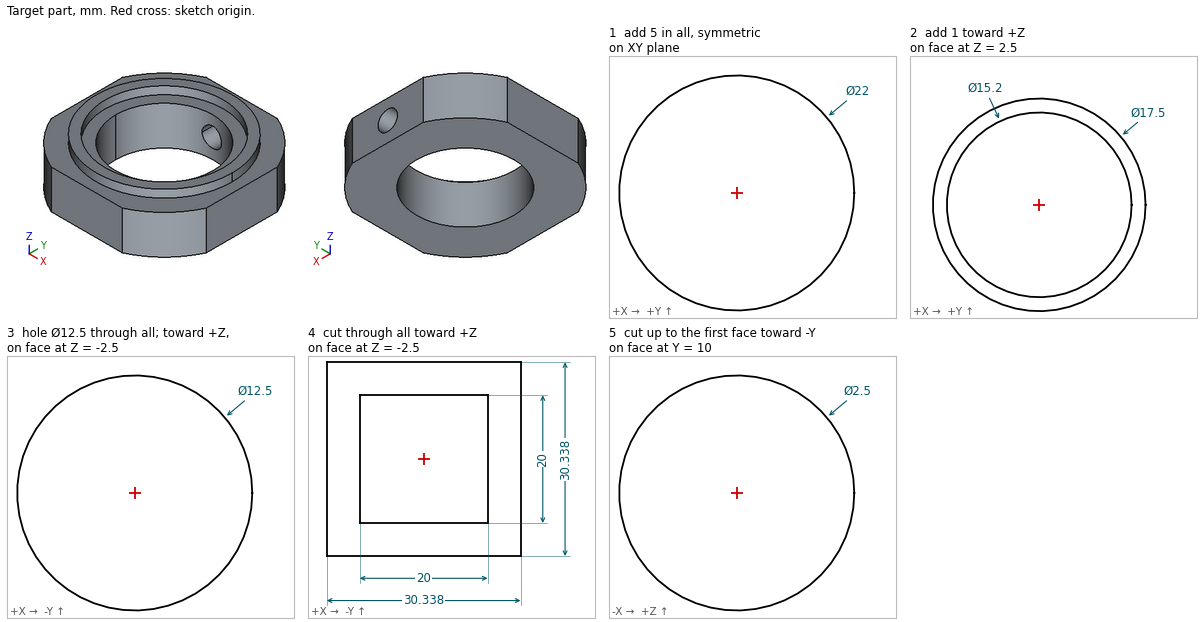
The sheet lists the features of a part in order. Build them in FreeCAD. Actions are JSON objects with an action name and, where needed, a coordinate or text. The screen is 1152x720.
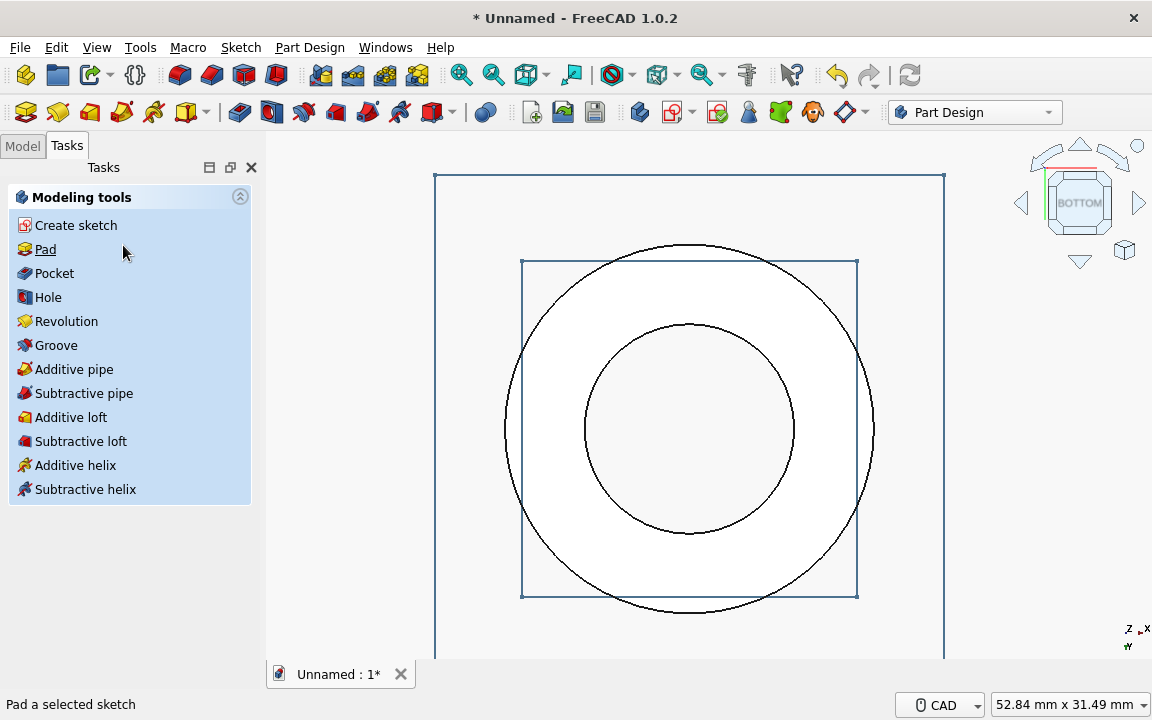
{"action": "left_click", "coordinate": [240, 112]}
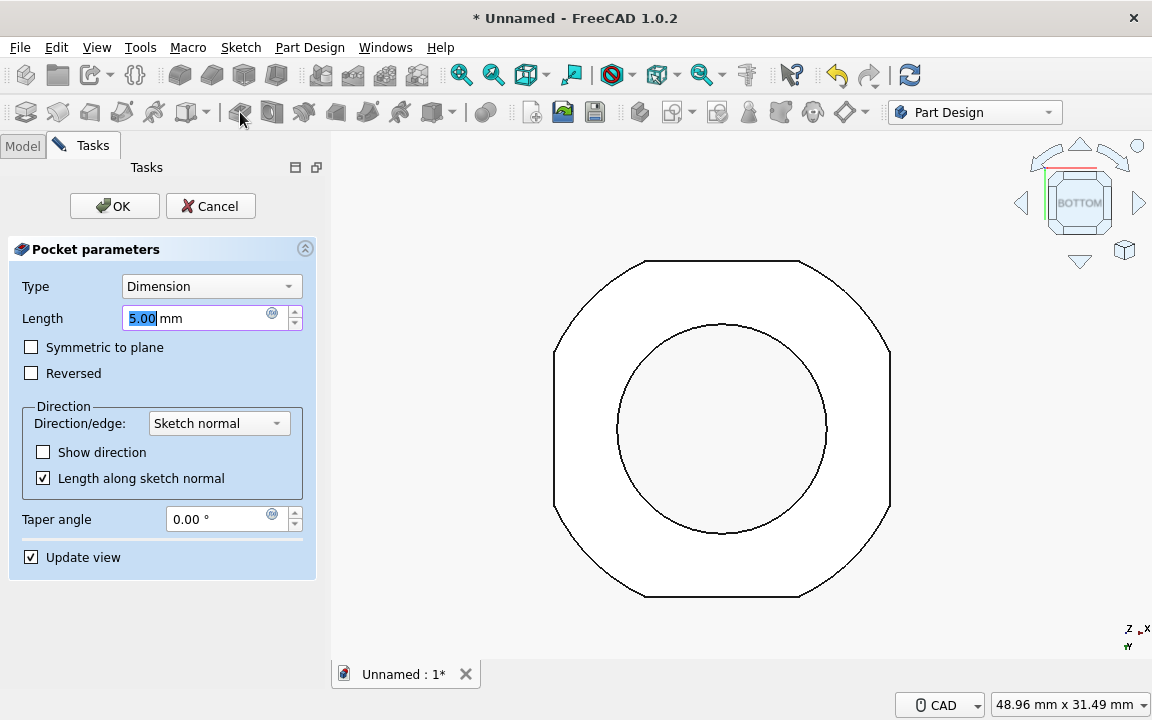
{"action": "left_click", "coordinate": [212, 286]}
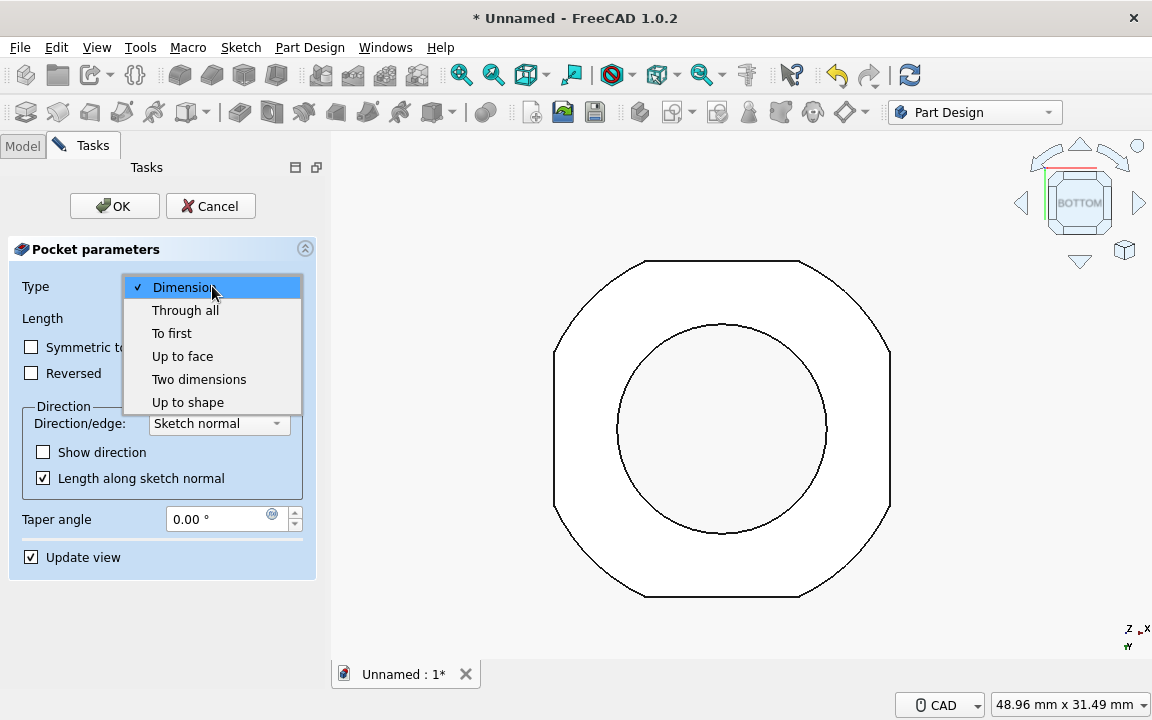
{"action": "left_click", "coordinate": [212, 310]}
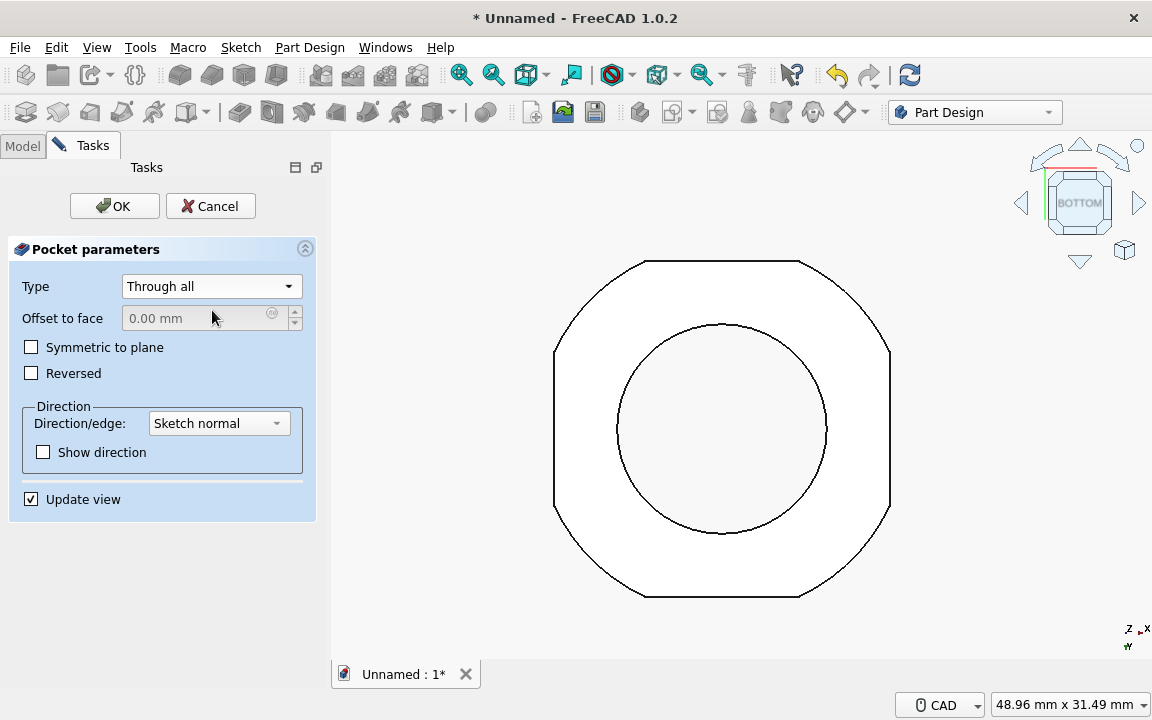
{"action": "left_click", "coordinate": [115, 206]}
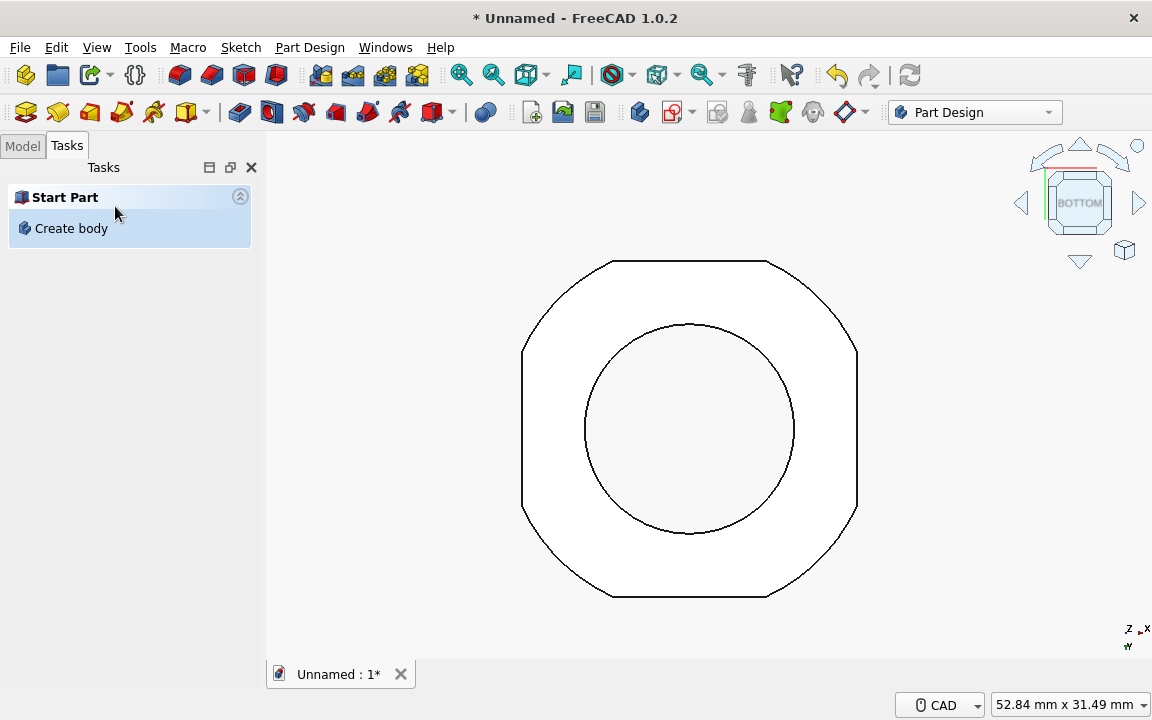
{"action": "key", "text": "4"}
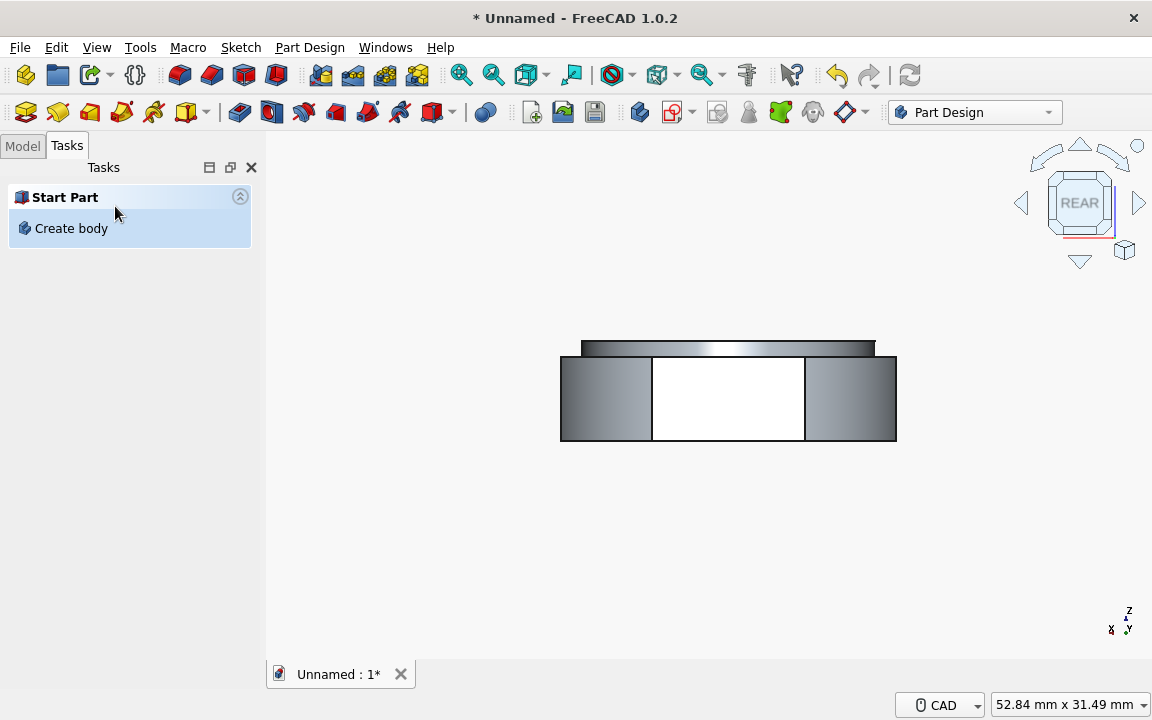
{"action": "key", "text": "v f"}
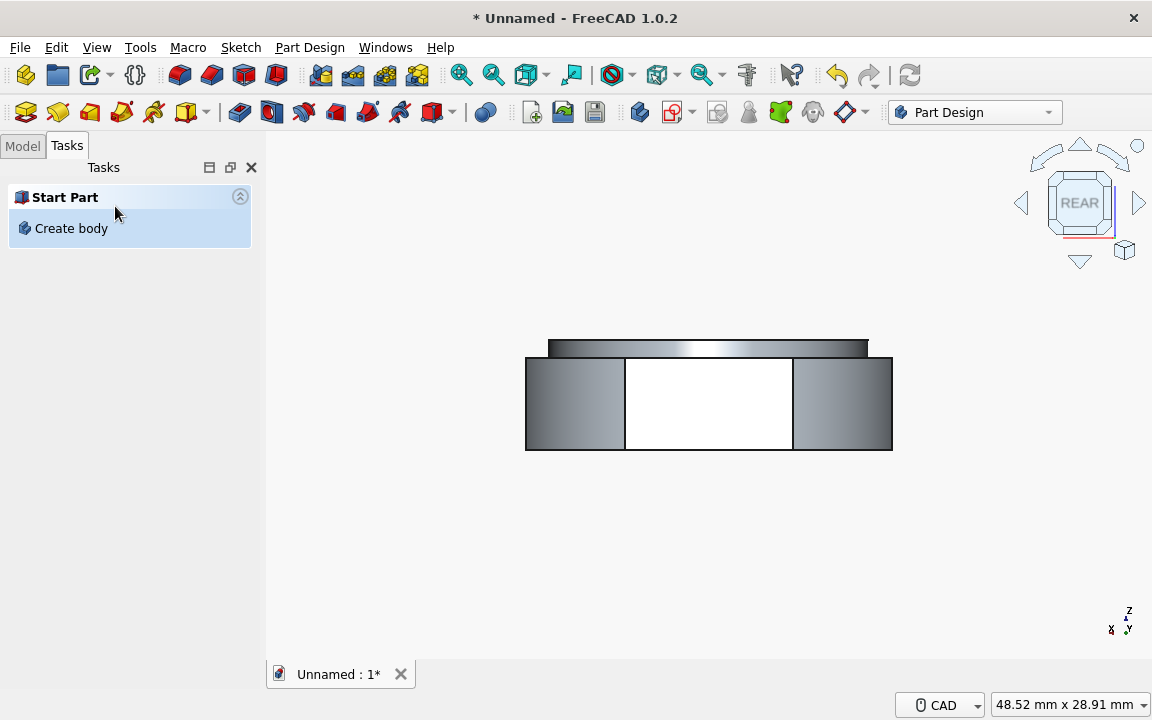
{"action": "left_click", "coordinate": [685, 403]}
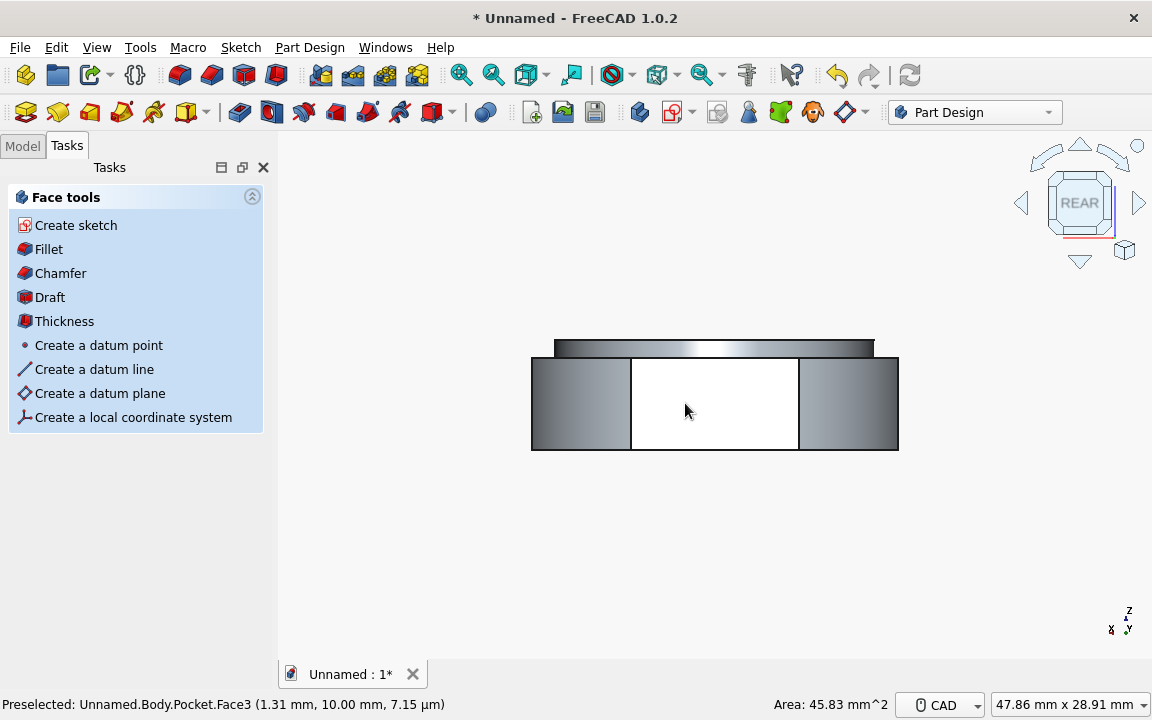
{"action": "left_click", "coordinate": [672, 112]}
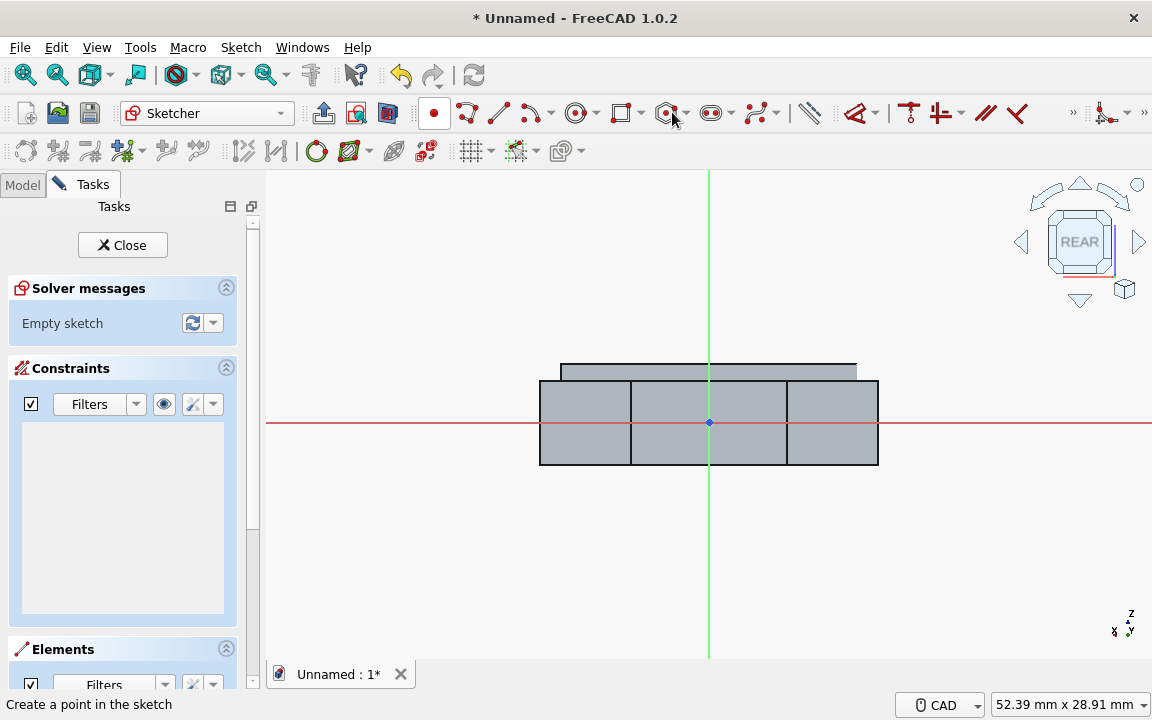
{"action": "scroll", "coordinate": [720, 424], "scroll_direction": "up", "scroll_amount": 10}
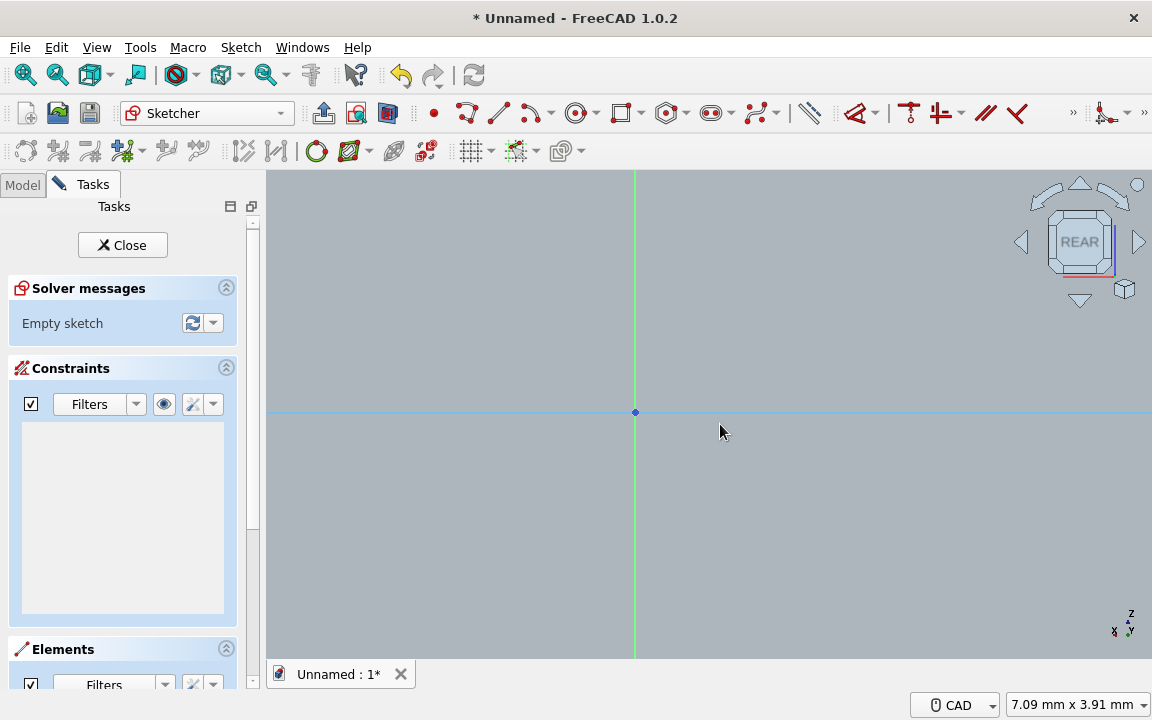
{"action": "left_click", "coordinate": [576, 114]}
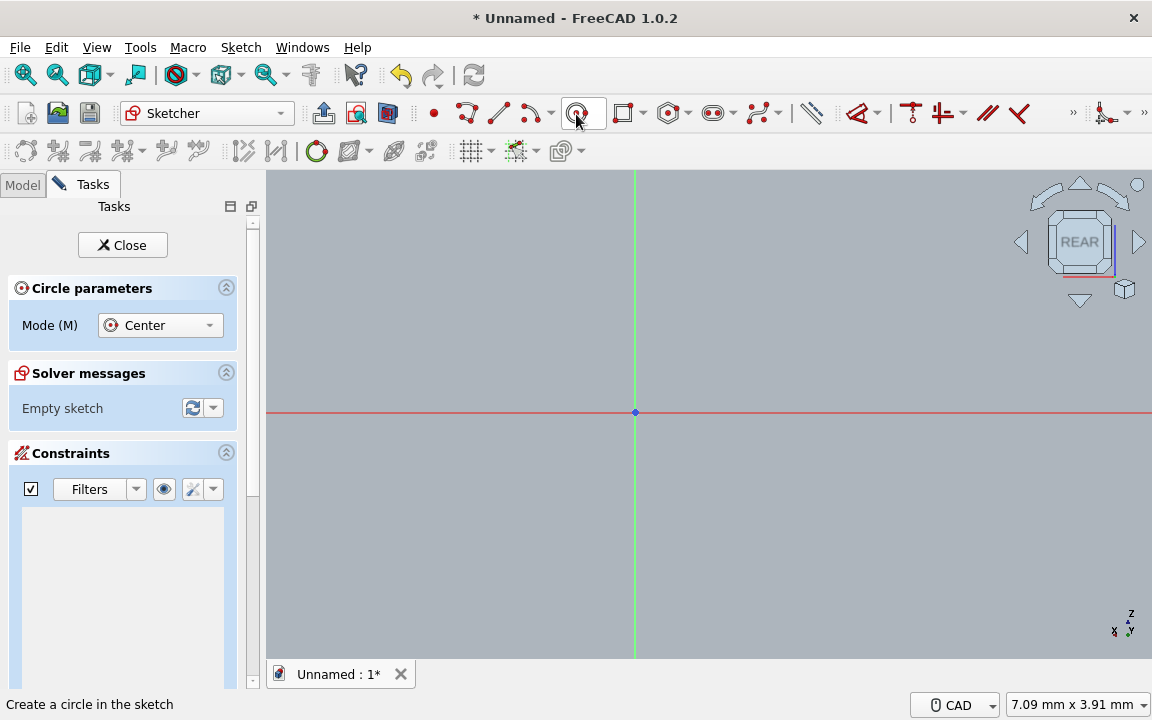
{"action": "left_click", "coordinate": [635, 413]}
{"action": "mouse_move", "coordinate": [746, 303]}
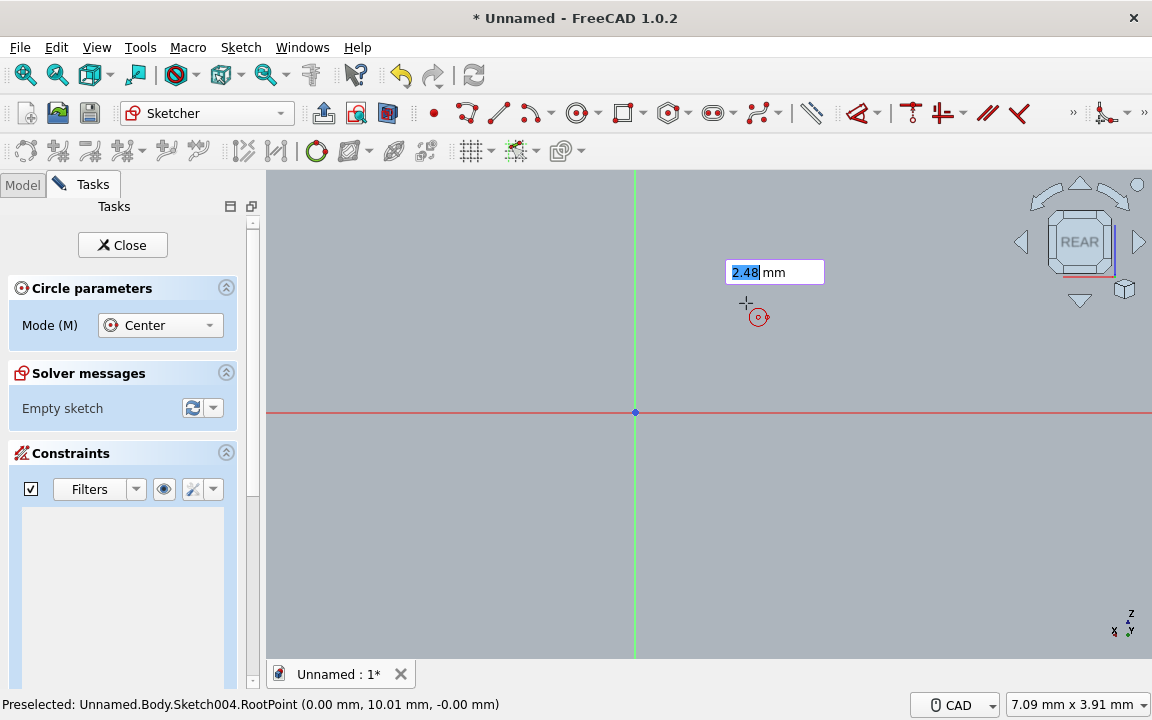
{"action": "type", "text": "2.5"}
{"action": "key", "text": "Return"}
{"action": "key", "text": "Escape"}